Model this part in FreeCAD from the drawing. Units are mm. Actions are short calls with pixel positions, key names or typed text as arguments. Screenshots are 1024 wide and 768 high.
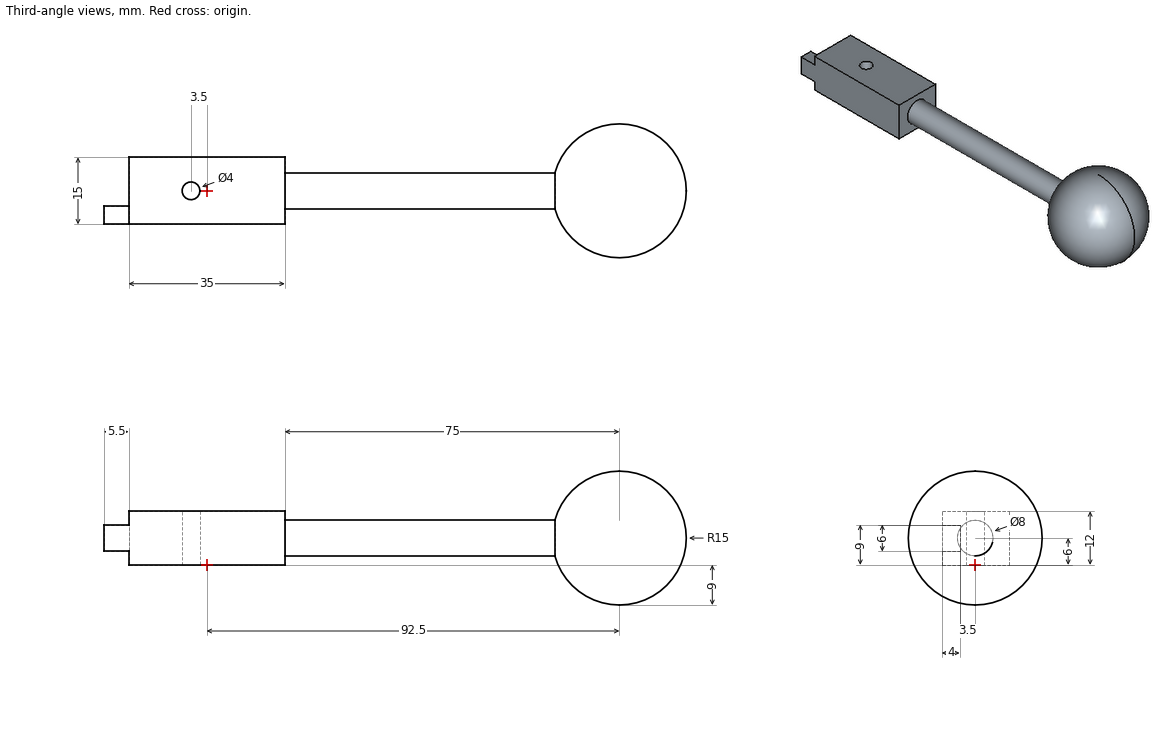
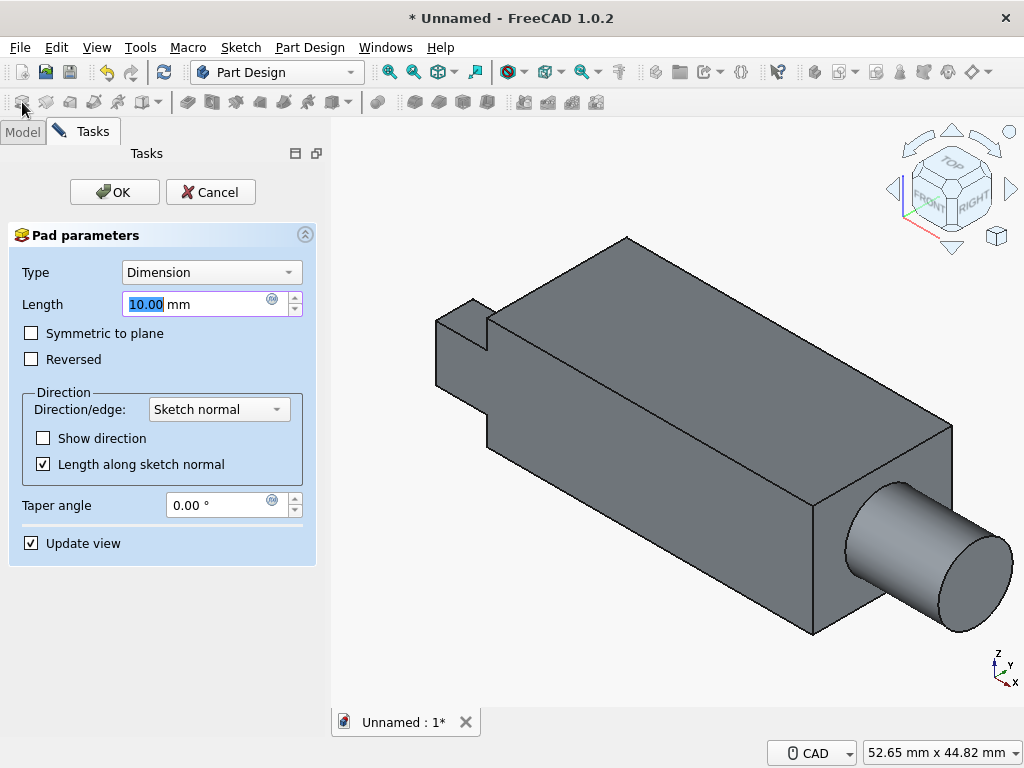
text(75)
key(Tab)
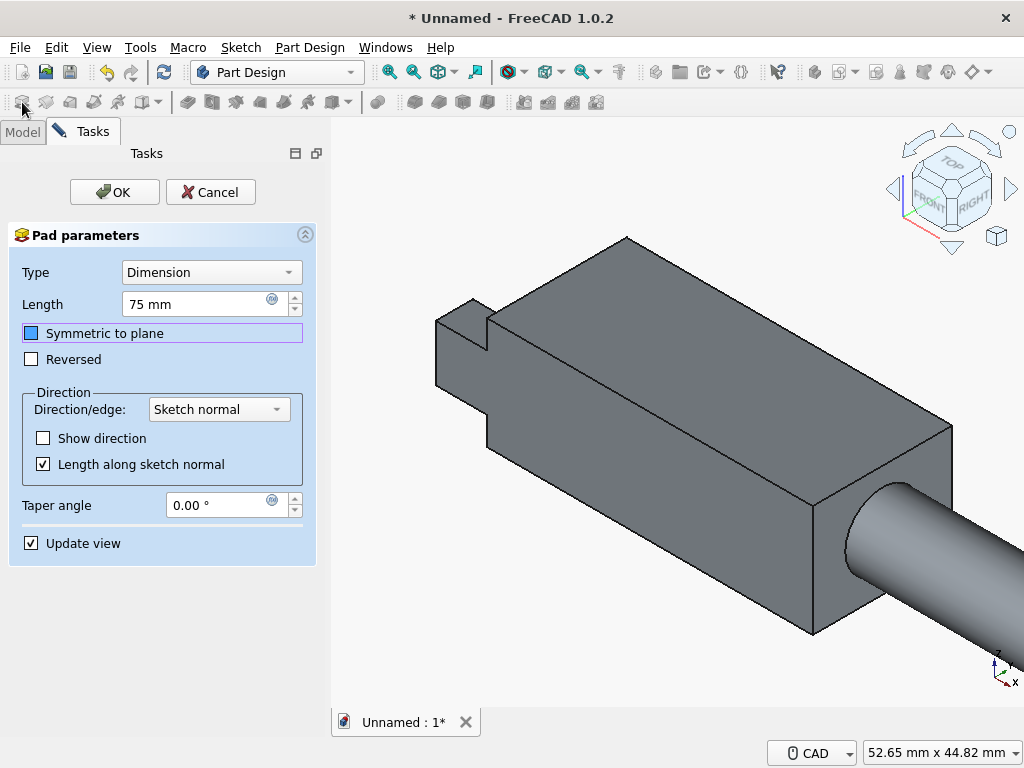
click(115, 192)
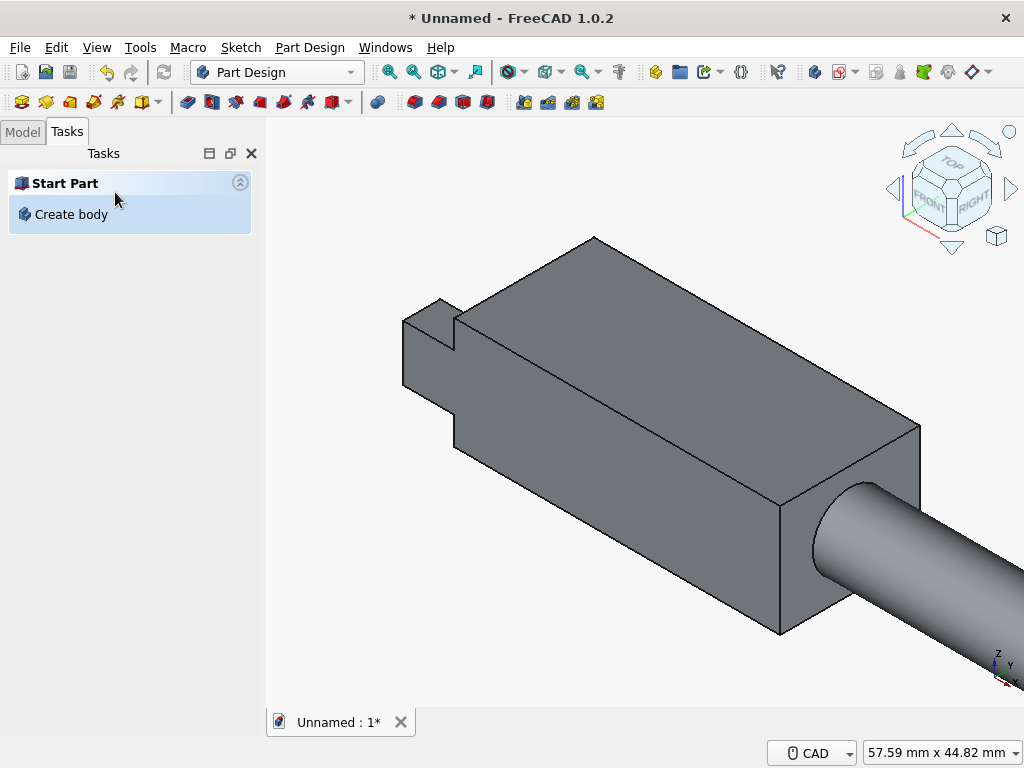
click(390, 72)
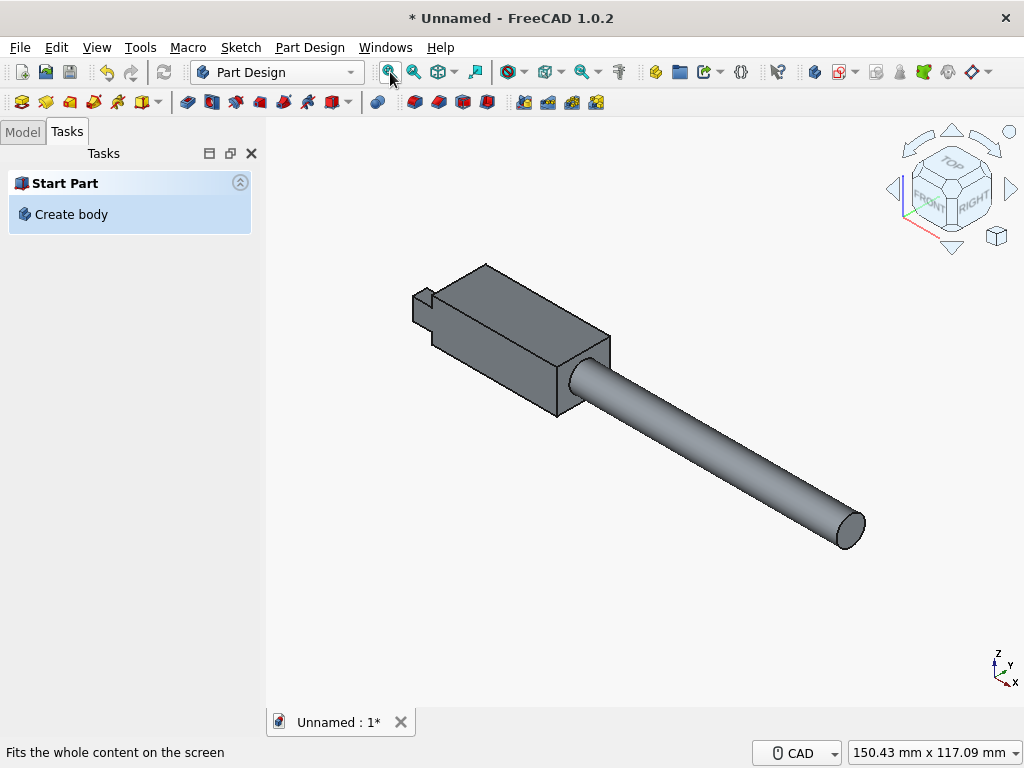
click(840, 72)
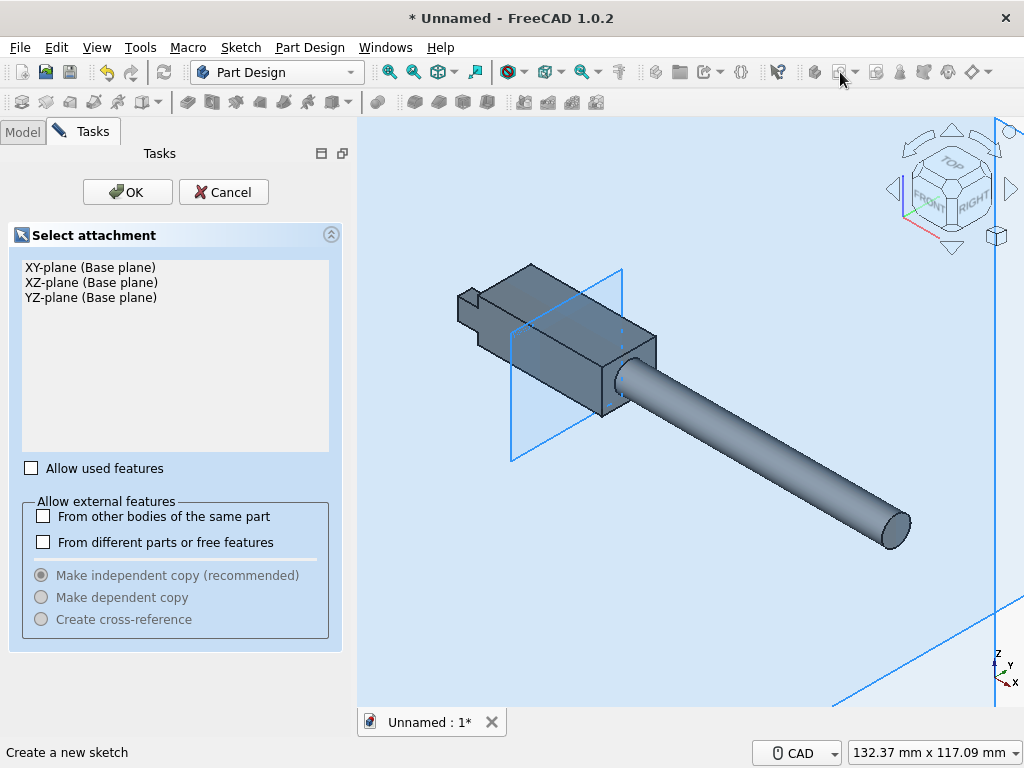
click(82, 282)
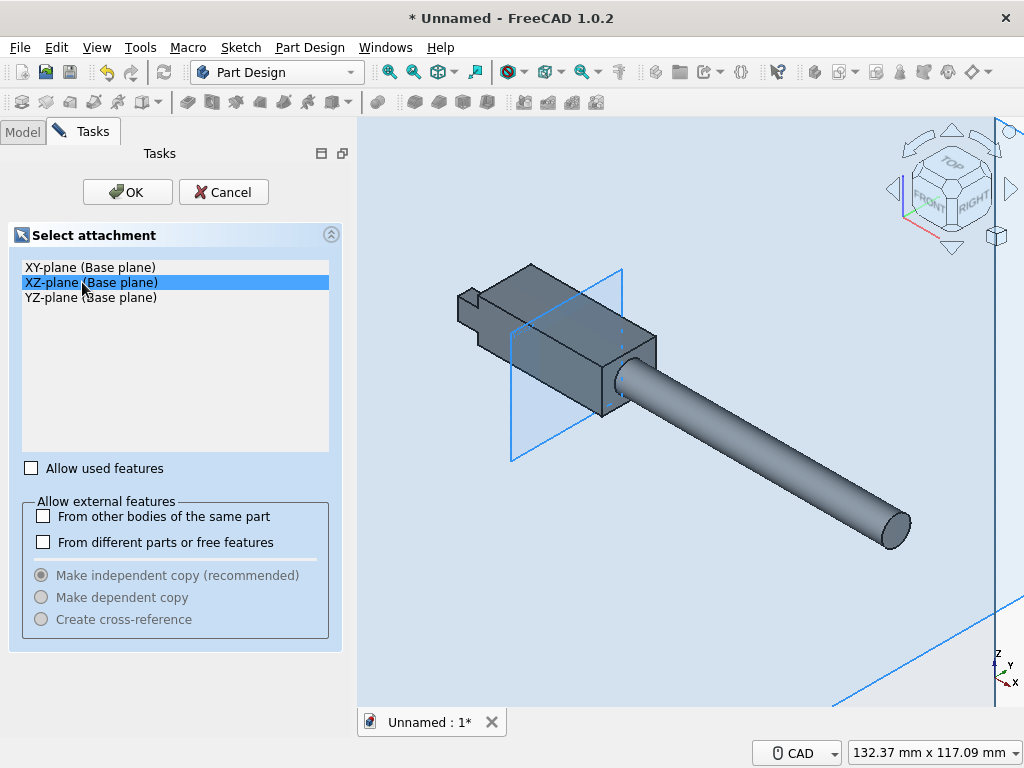
click(128, 192)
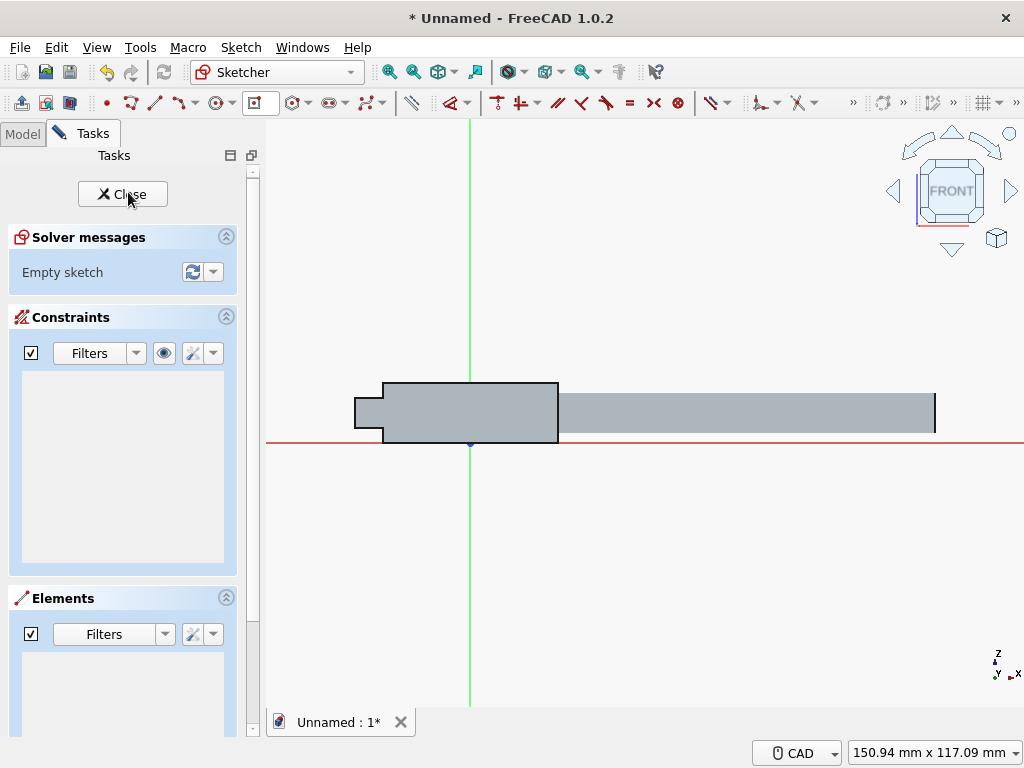
click(70, 104)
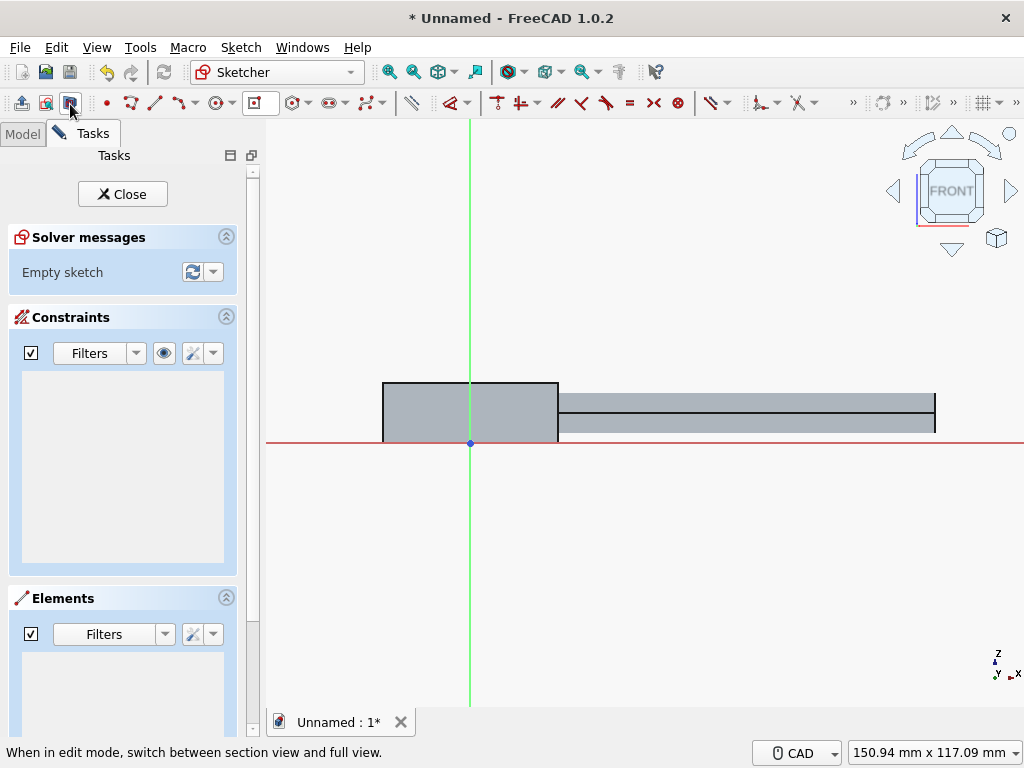
scroll(576, 413, down, 5)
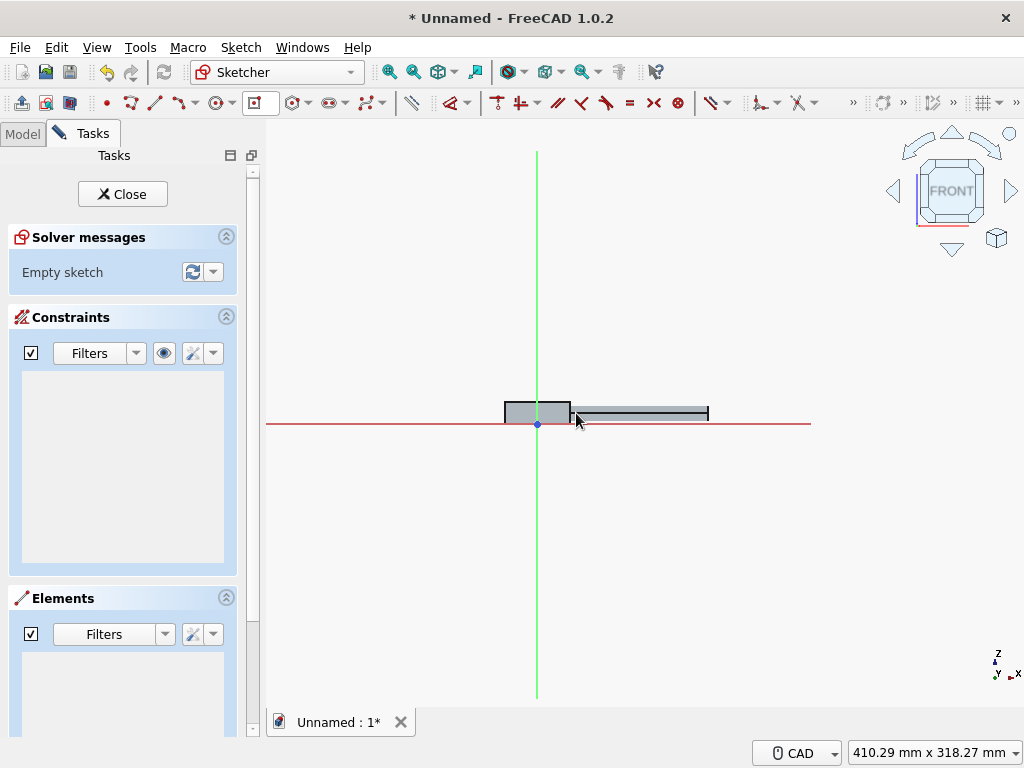
scroll(759, 400, up, 8)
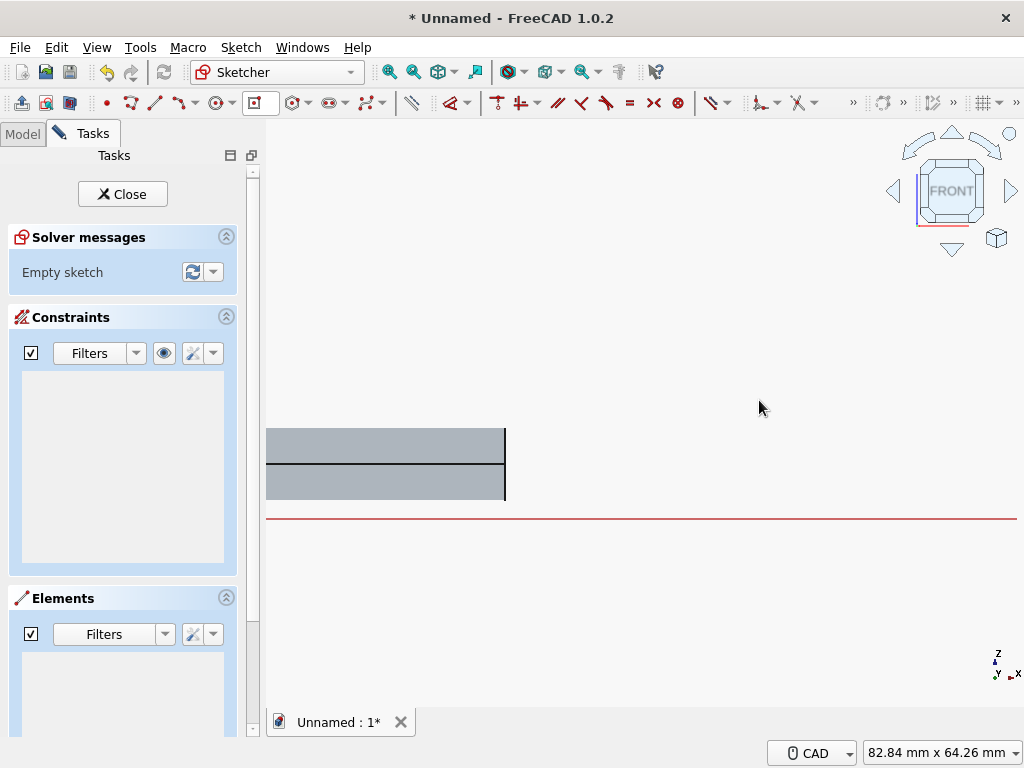
click(156, 104)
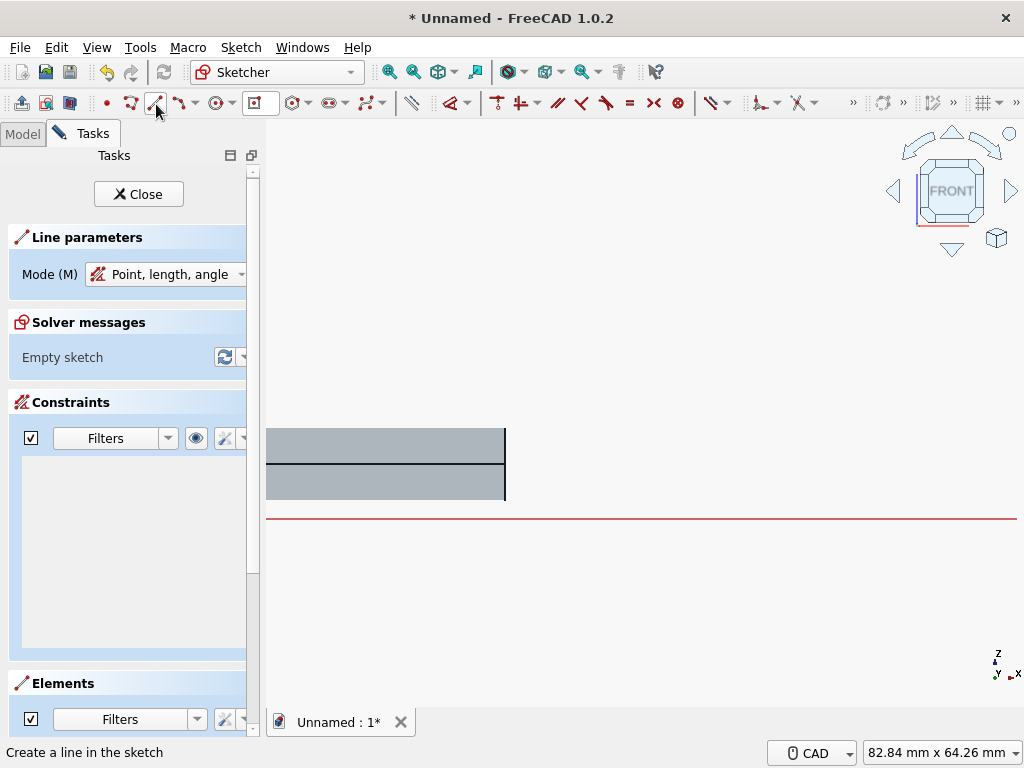
click(505, 601)
click(505, 327)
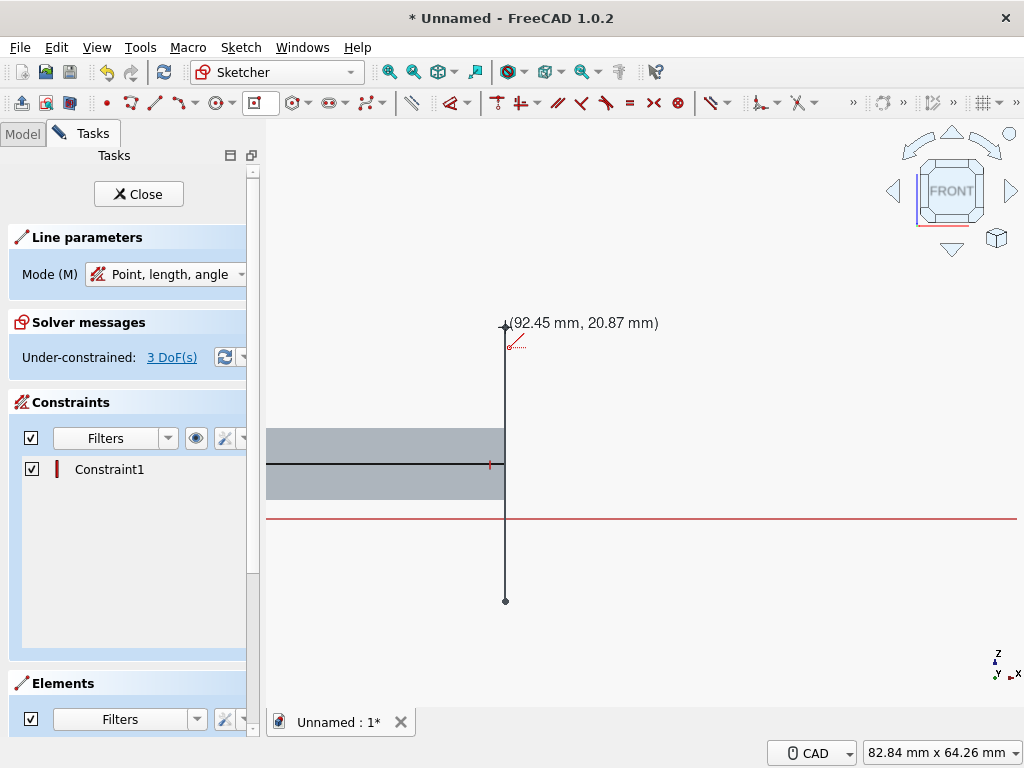
click(180, 104)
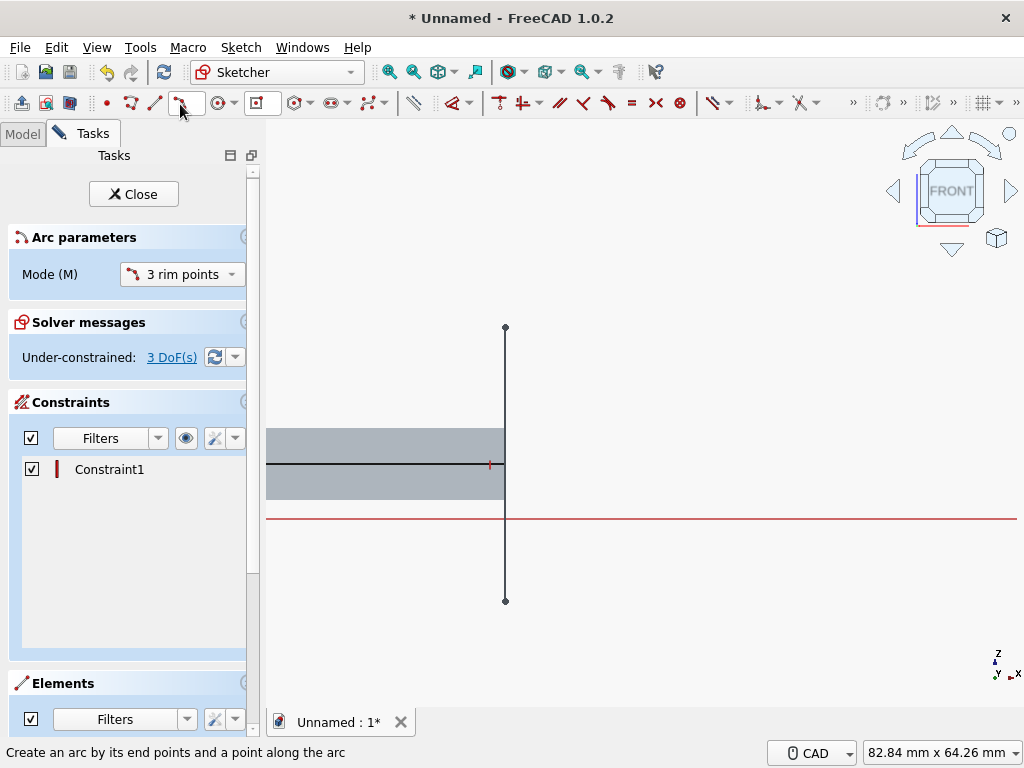
click(505, 328)
click(505, 602)
click(643, 464)